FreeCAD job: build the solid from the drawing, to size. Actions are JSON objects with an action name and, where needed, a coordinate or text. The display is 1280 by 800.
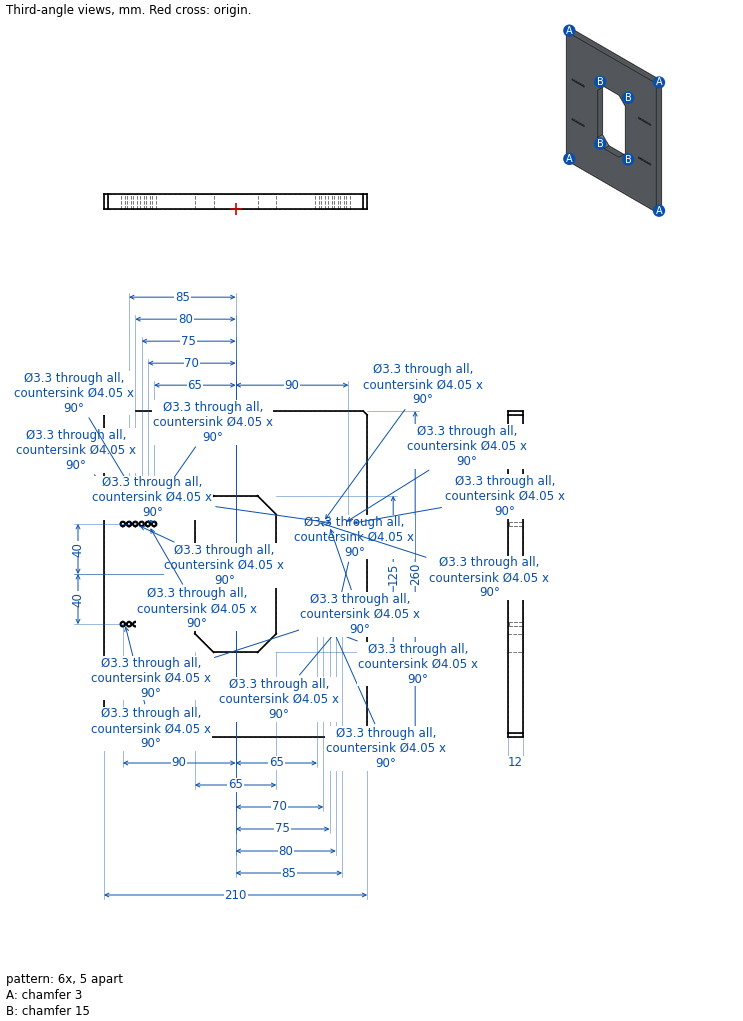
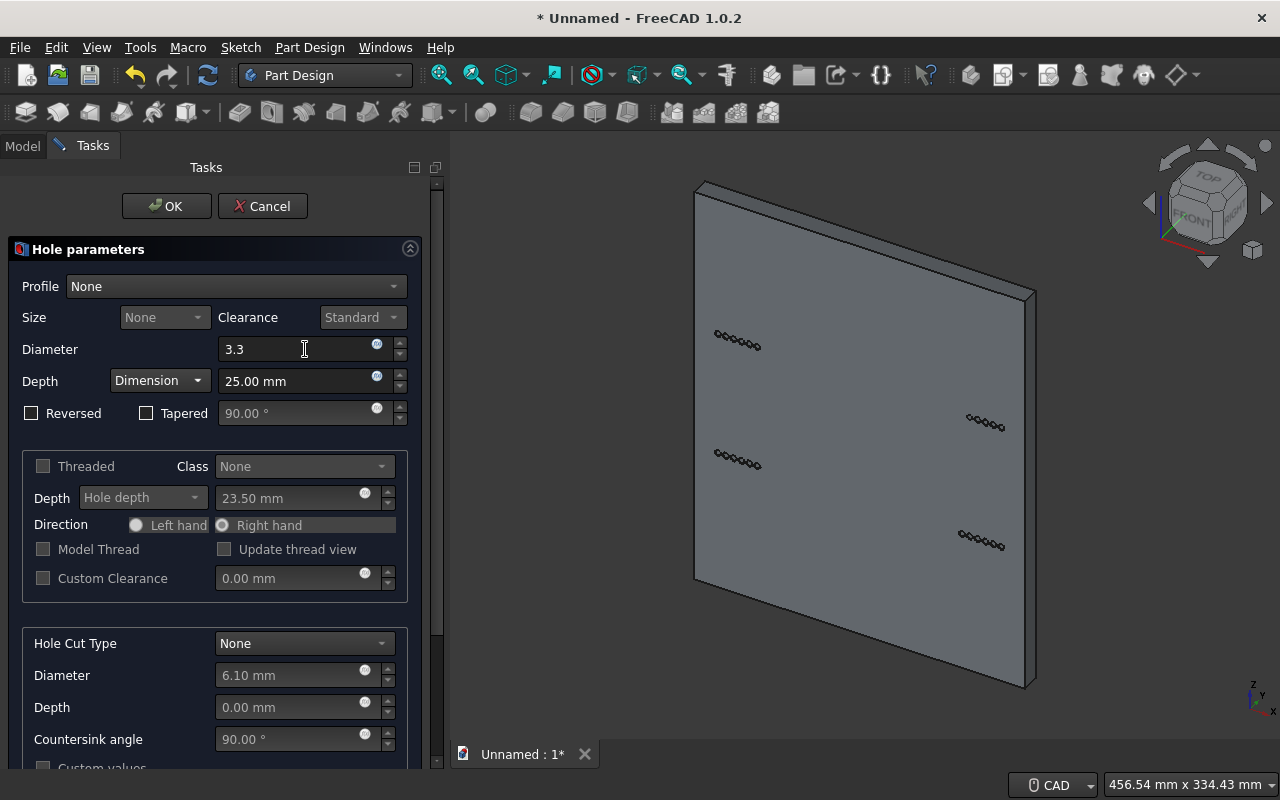
{"action": "left_click", "coordinate": [161, 380]}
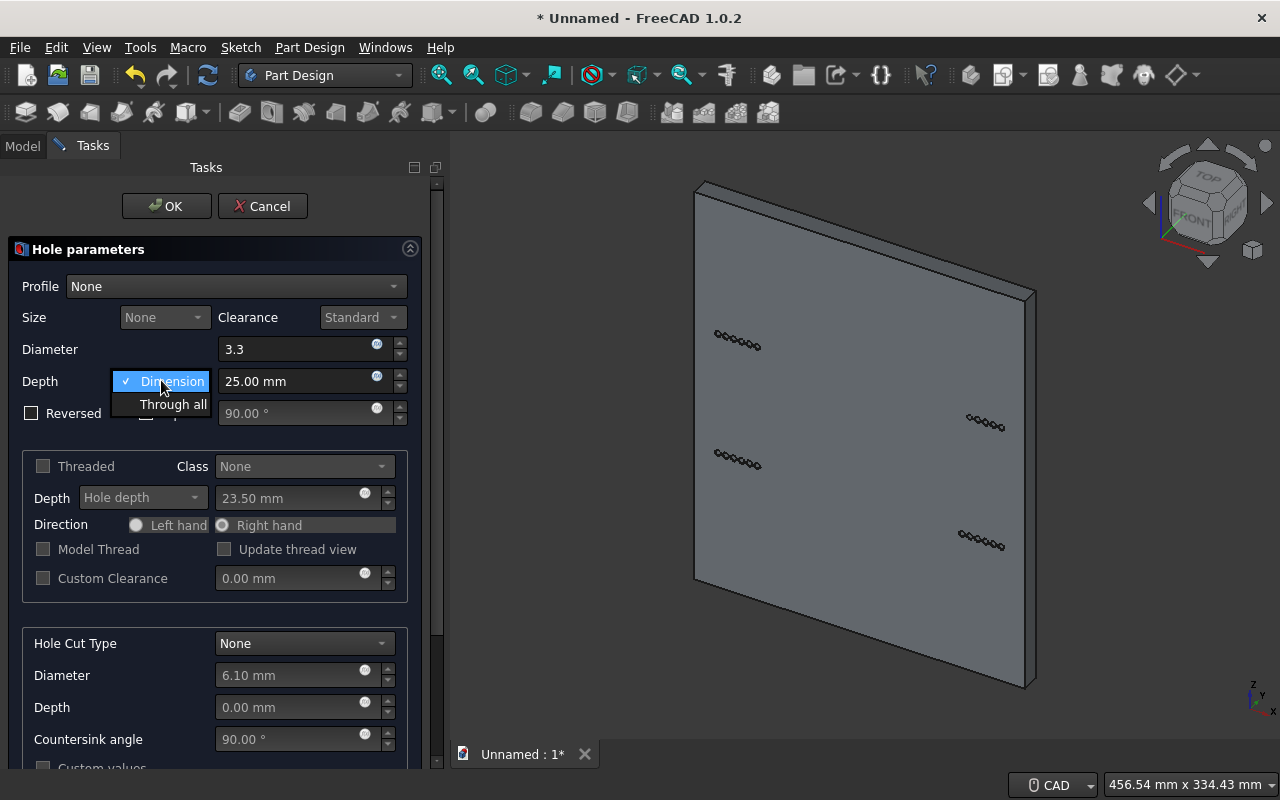
{"action": "left_click", "coordinate": [160, 404]}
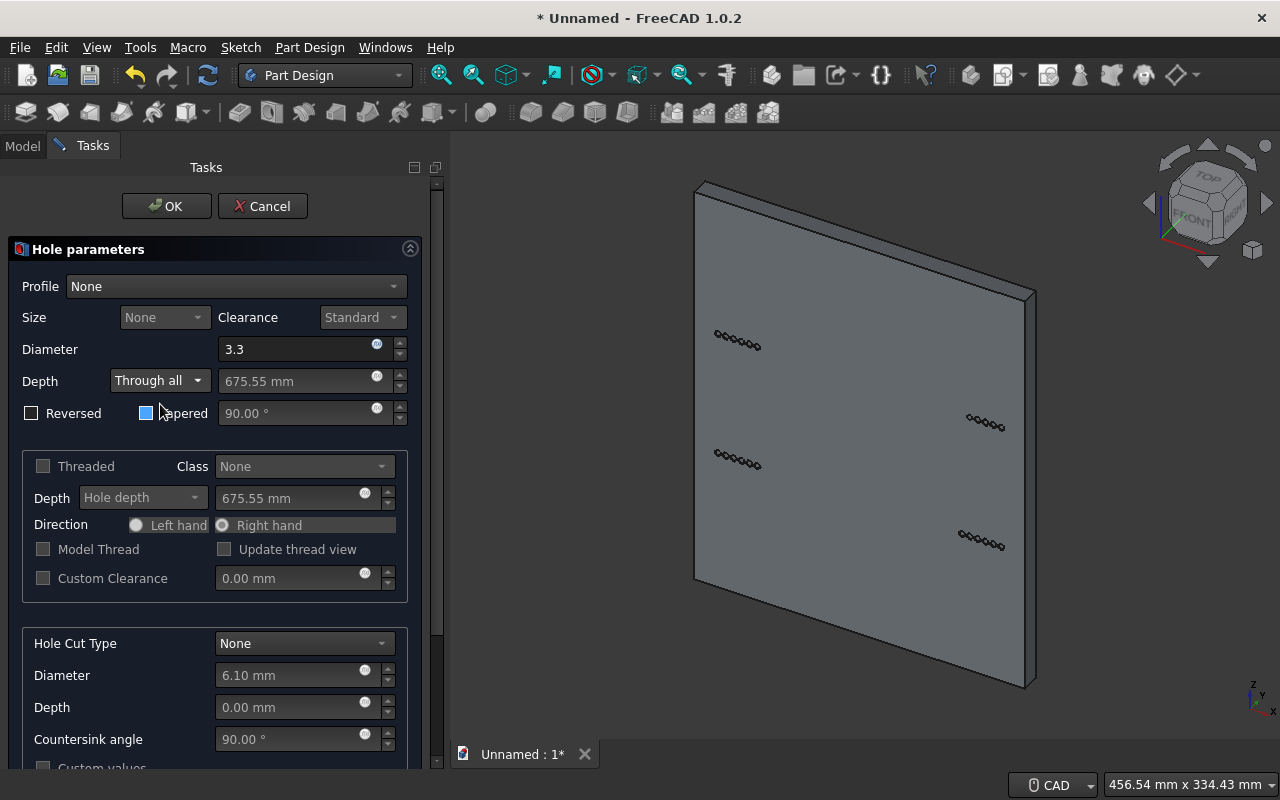
{"action": "left_click", "coordinate": [306, 644]}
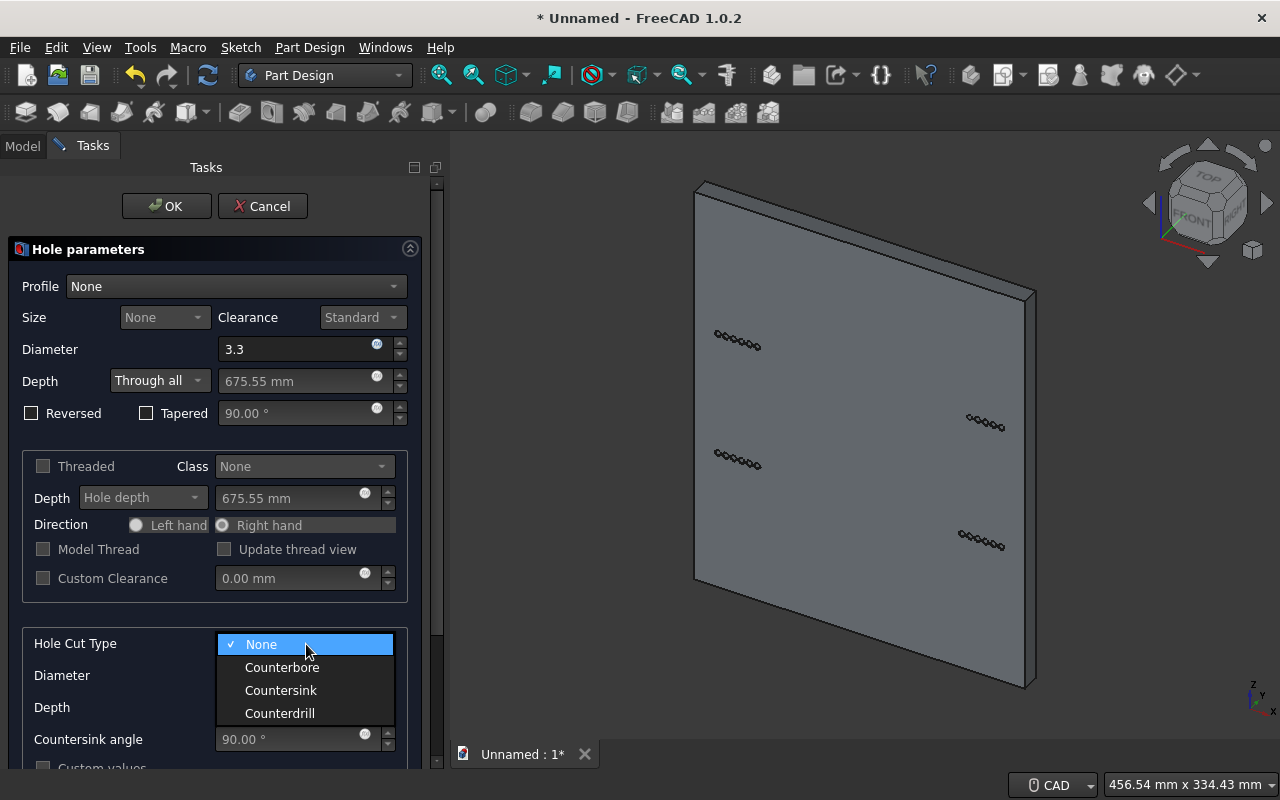
{"action": "left_click", "coordinate": [304, 690]}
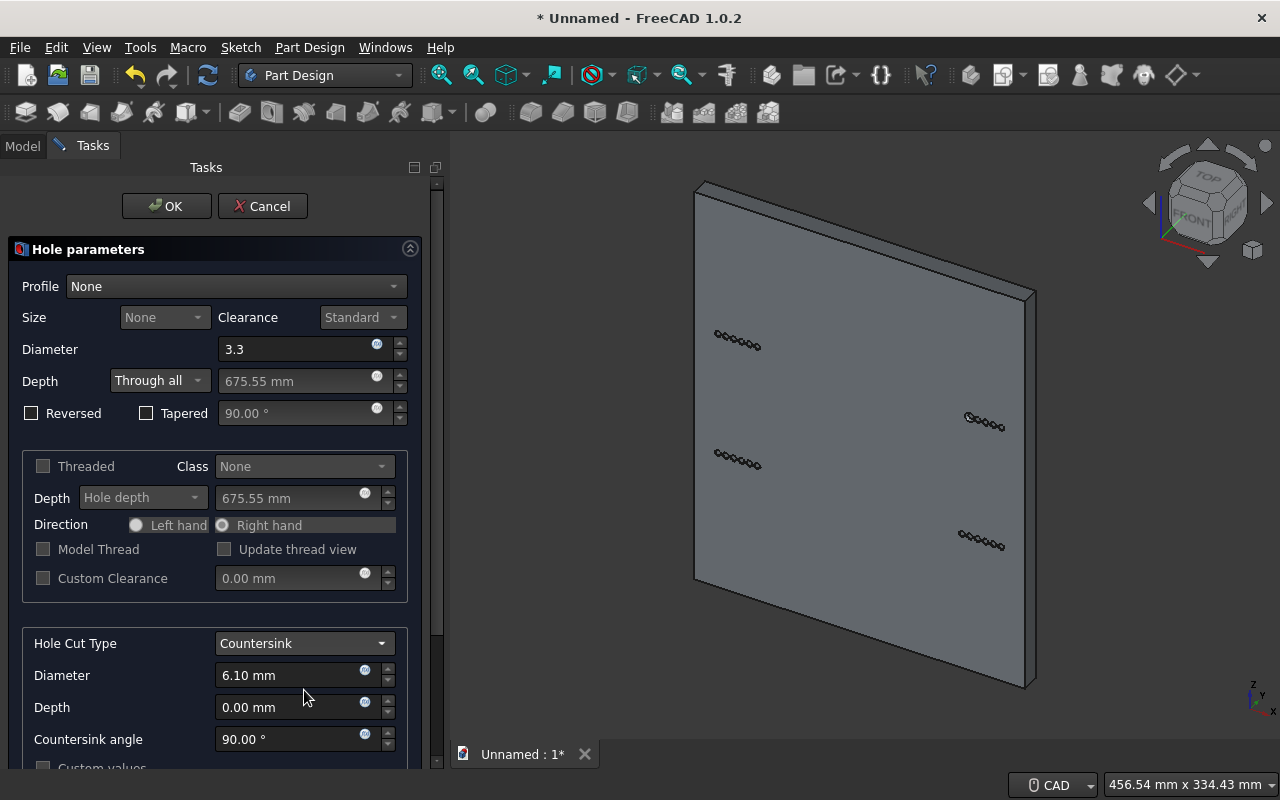
{"action": "triple_click", "coordinate": [298, 675]}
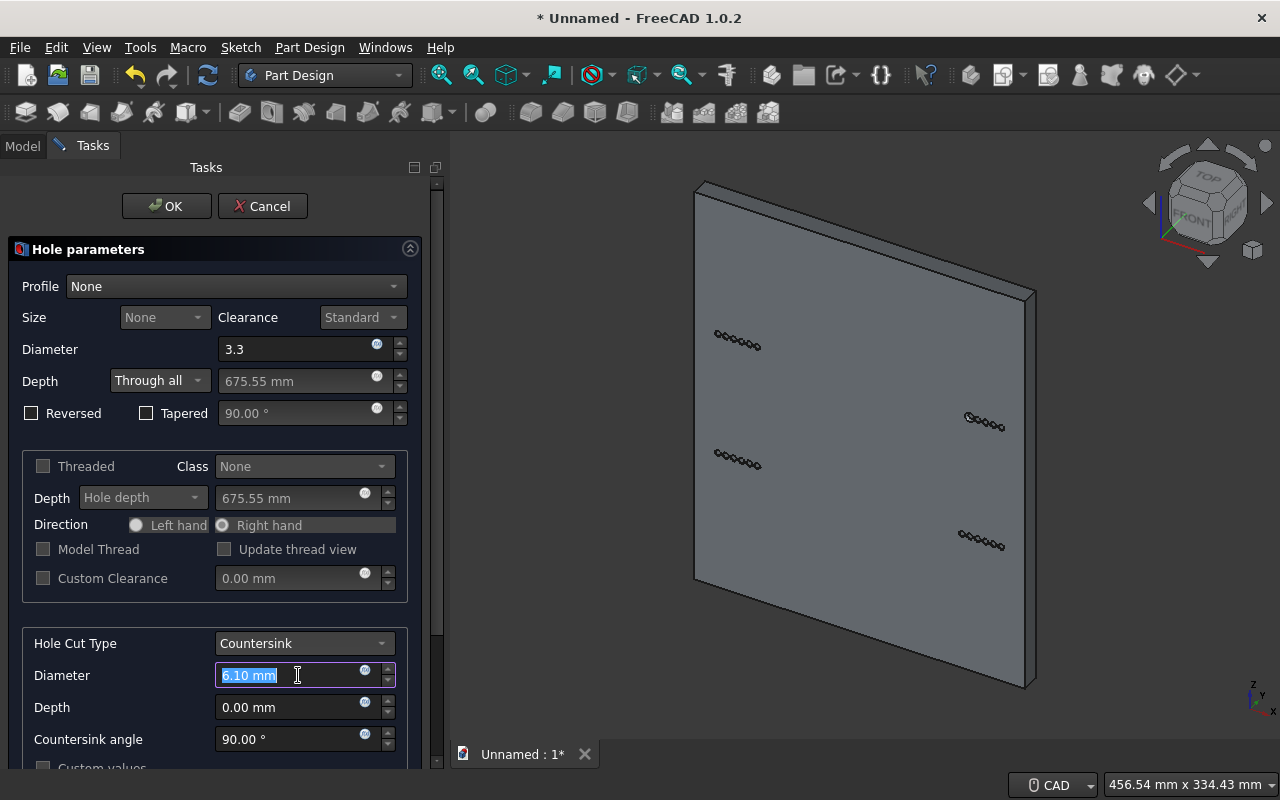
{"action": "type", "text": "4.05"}
{"action": "key", "text": "Tab"}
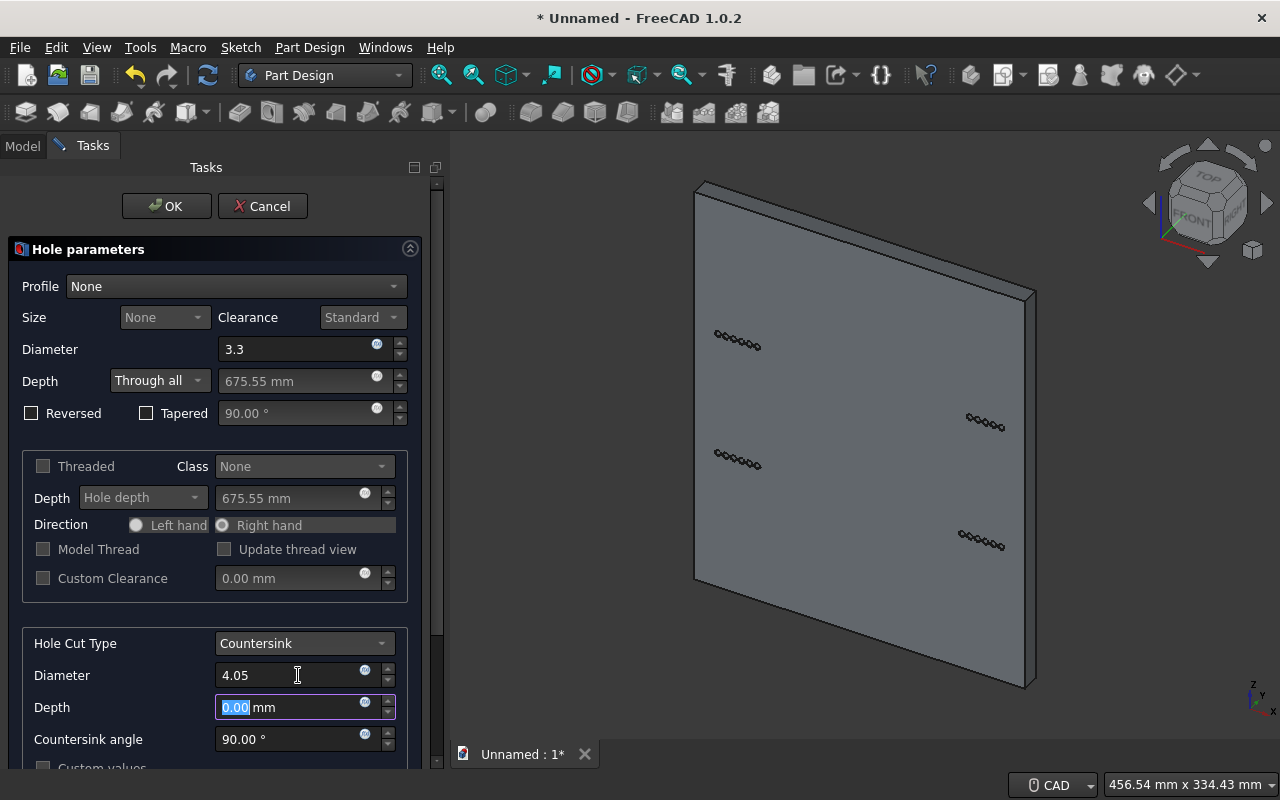
{"action": "left_click", "coordinate": [167, 206]}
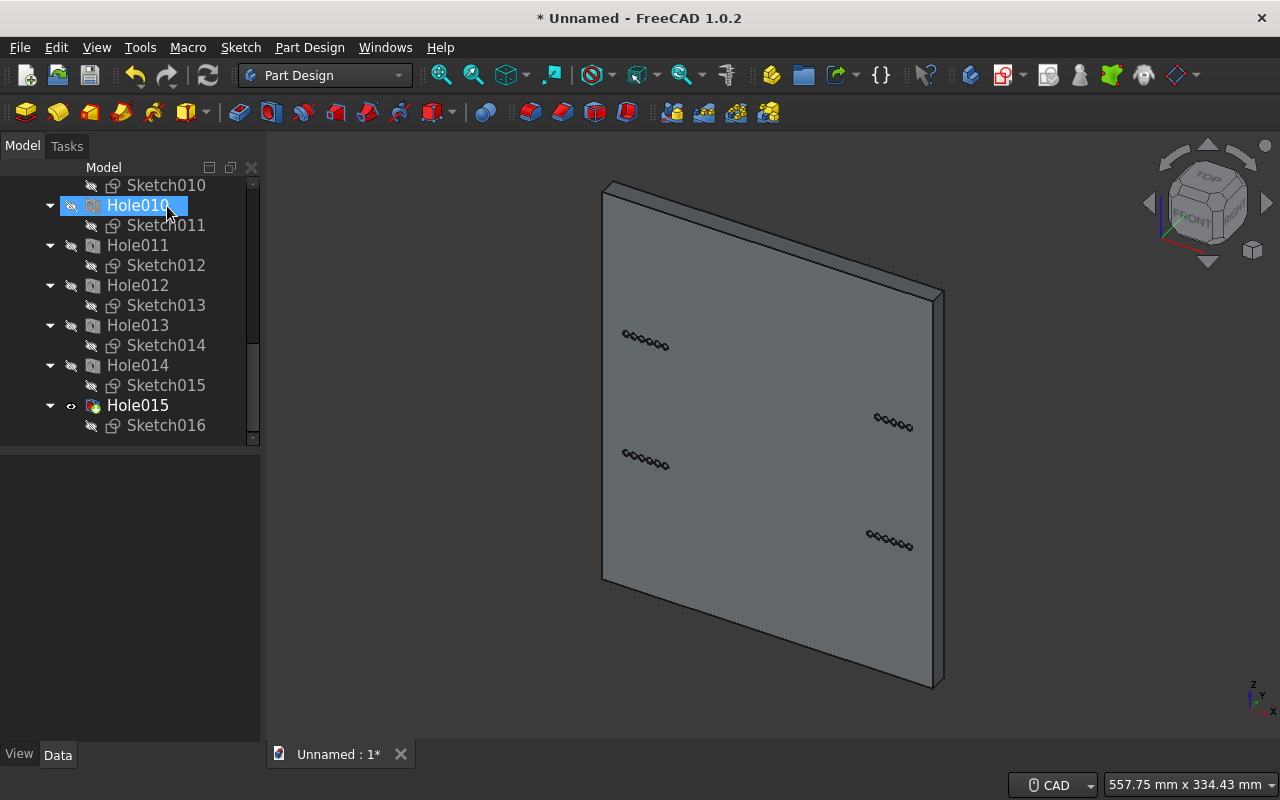
{"action": "left_click", "coordinate": [768, 439]}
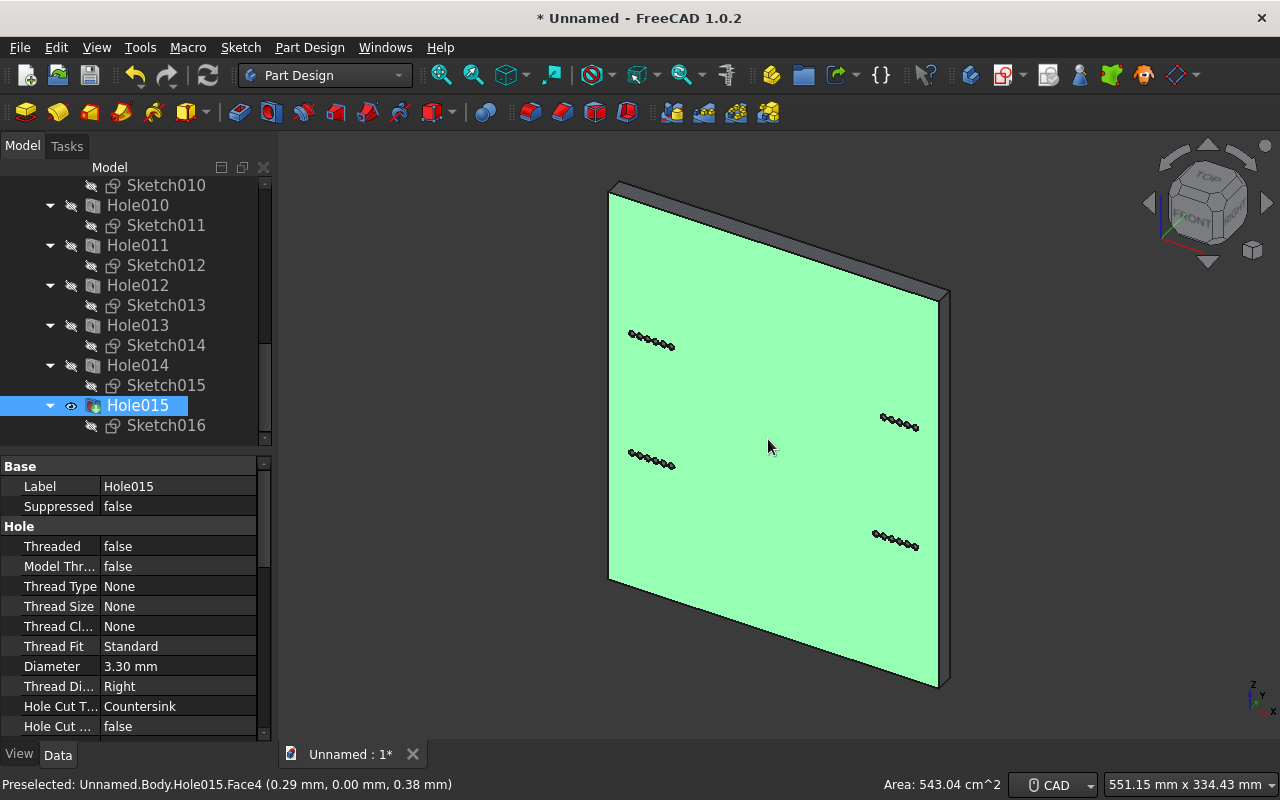
{"action": "left_click", "coordinate": [1004, 76]}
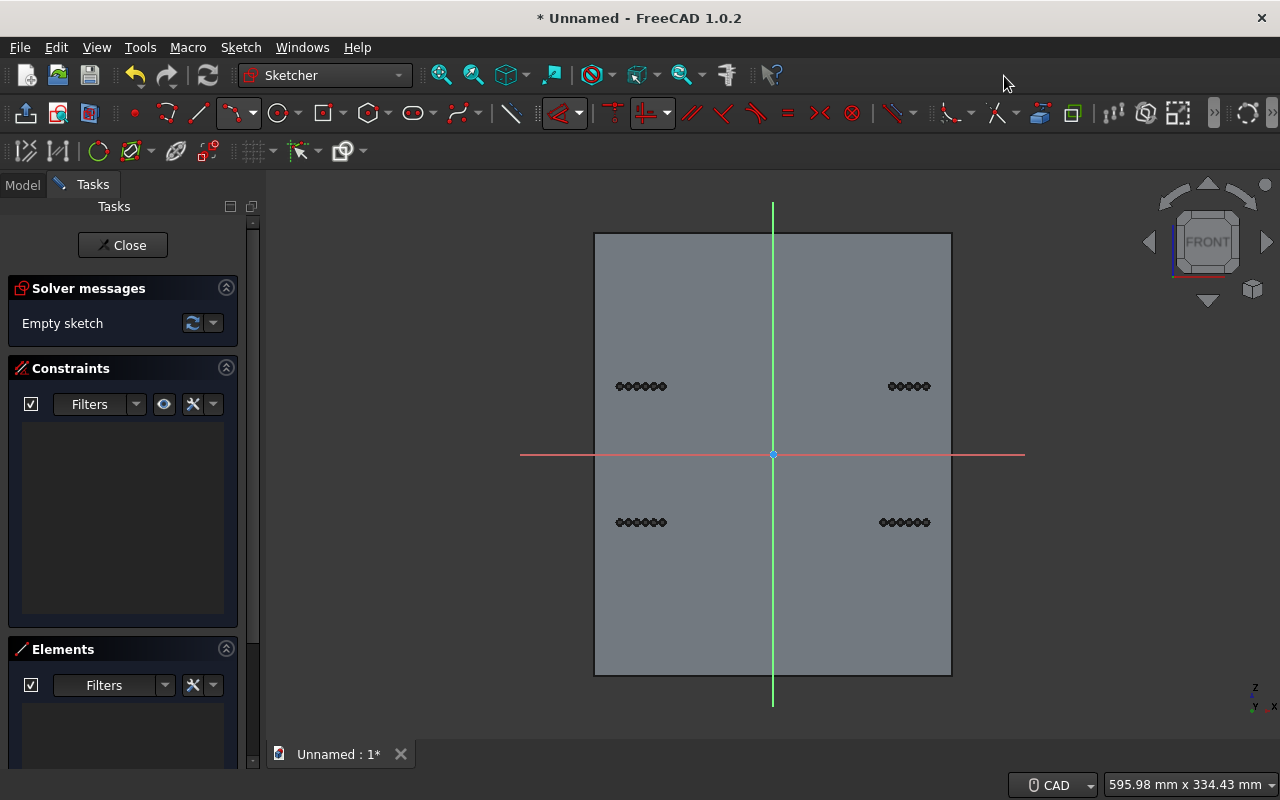
{"action": "scroll", "coordinate": [893, 383], "scroll_direction": "up", "scroll_amount": 15}